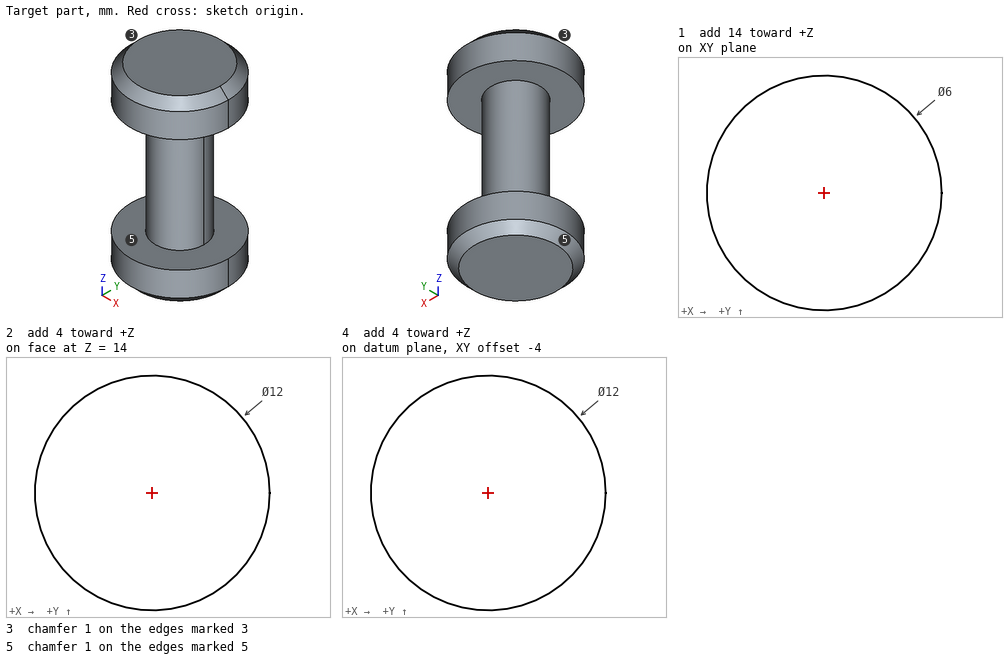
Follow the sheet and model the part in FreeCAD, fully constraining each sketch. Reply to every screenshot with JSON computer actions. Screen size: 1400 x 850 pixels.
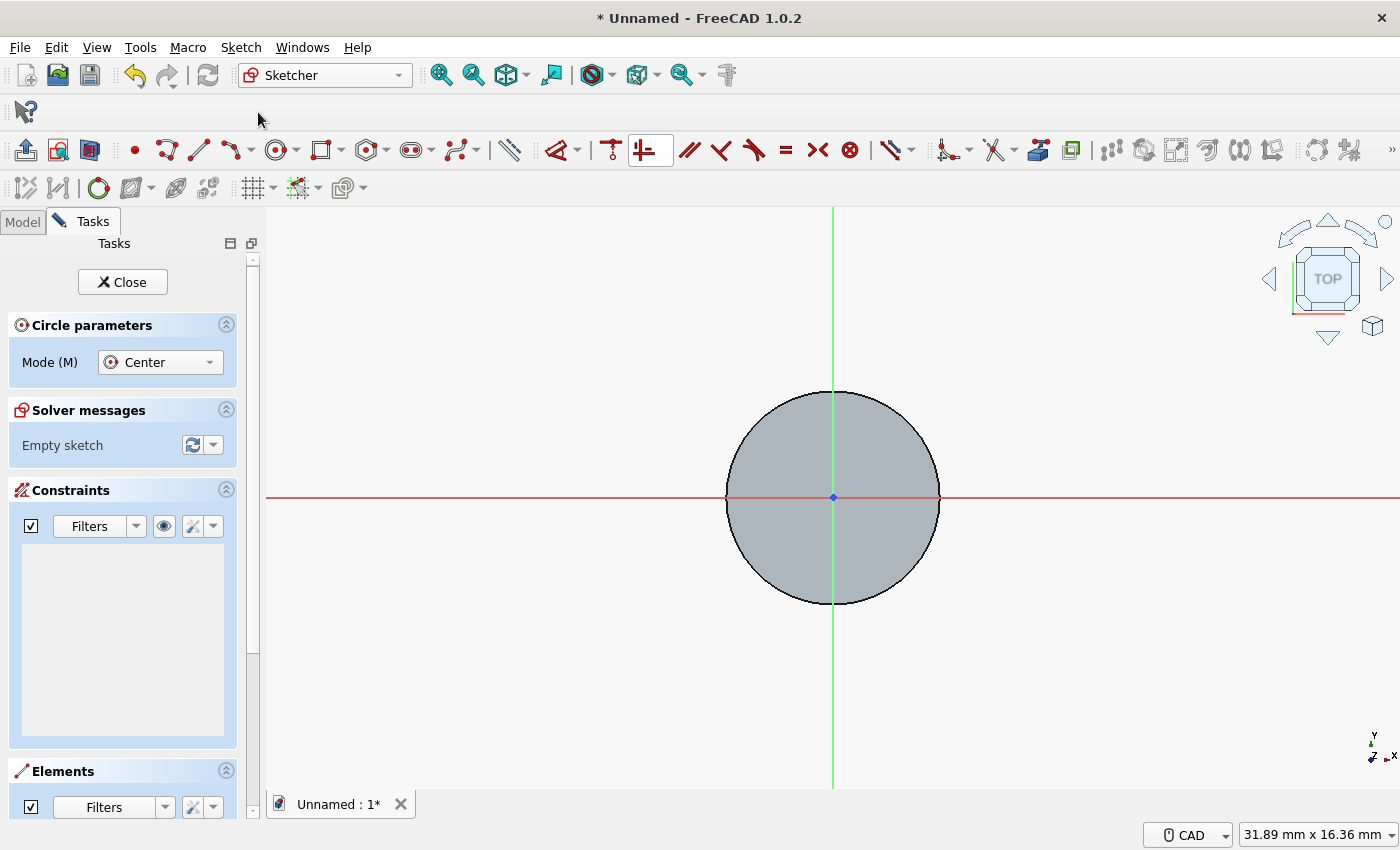
{"action": "left_click", "coordinate": [833, 498]}
{"action": "left_click", "coordinate": [984, 347]}
{"action": "key", "text": "Escape"}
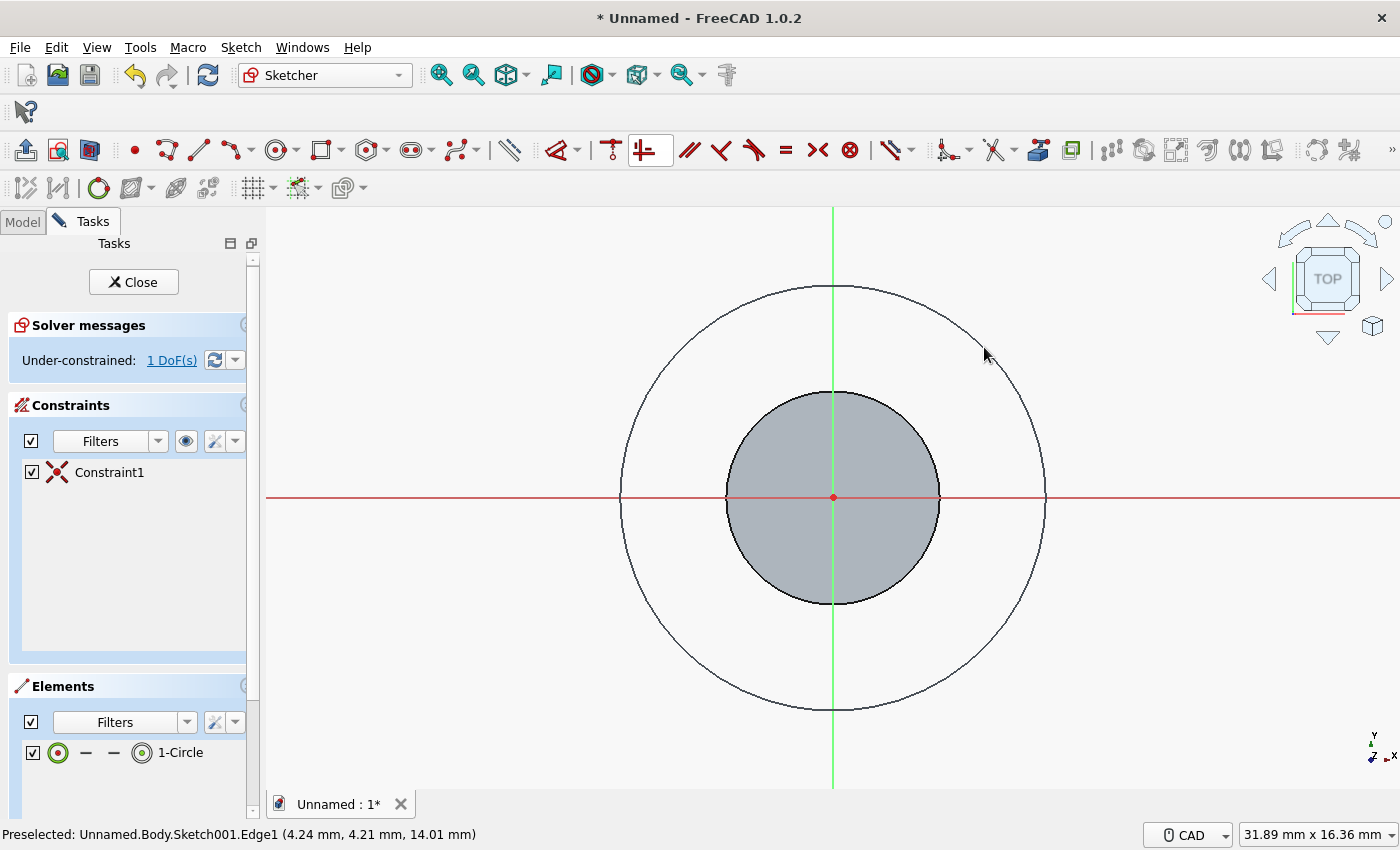
{"action": "left_click", "coordinate": [983, 347]}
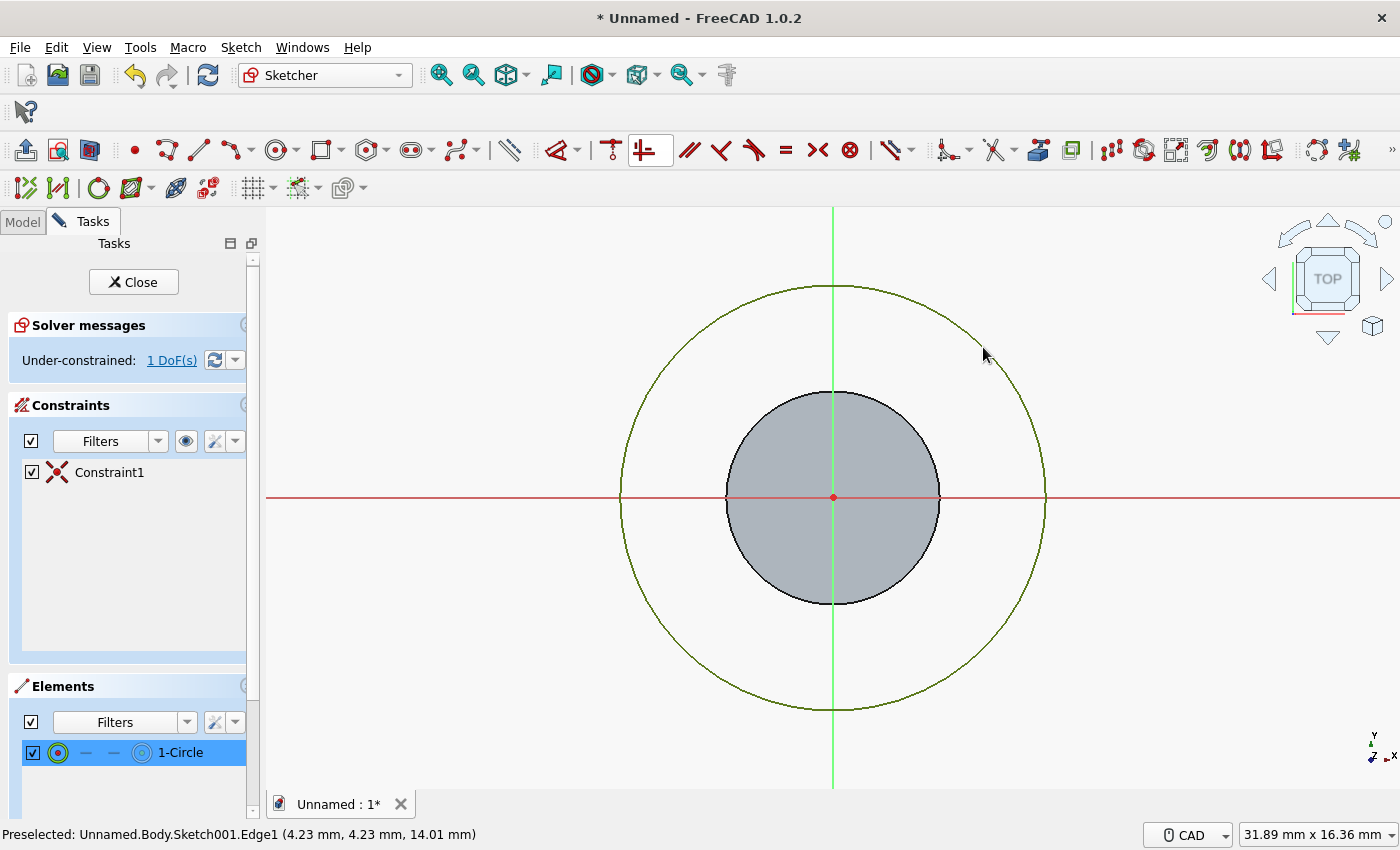
{"action": "key", "text": "k o"}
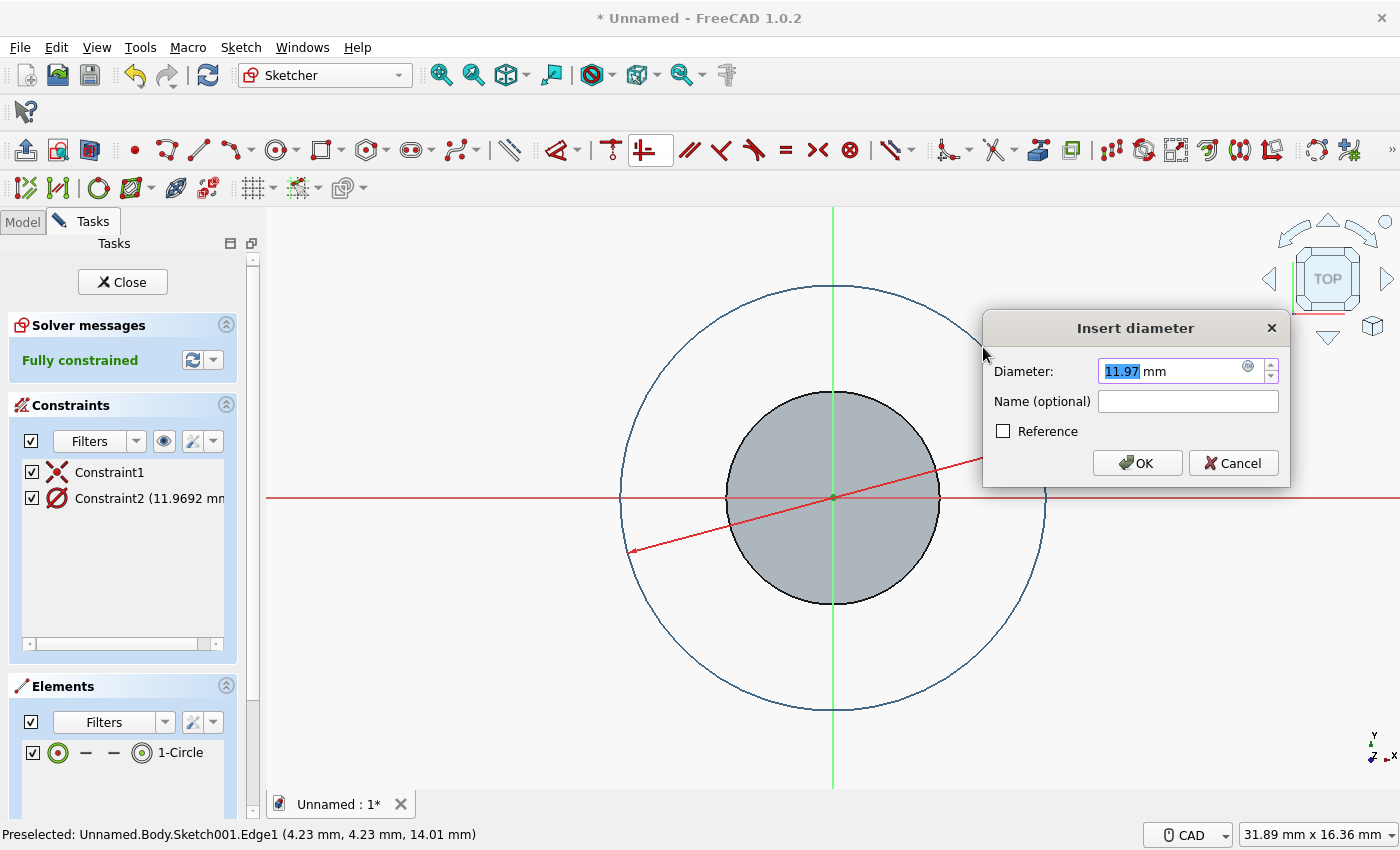
{"action": "type", "text": "12"}
{"action": "key", "text": "Return"}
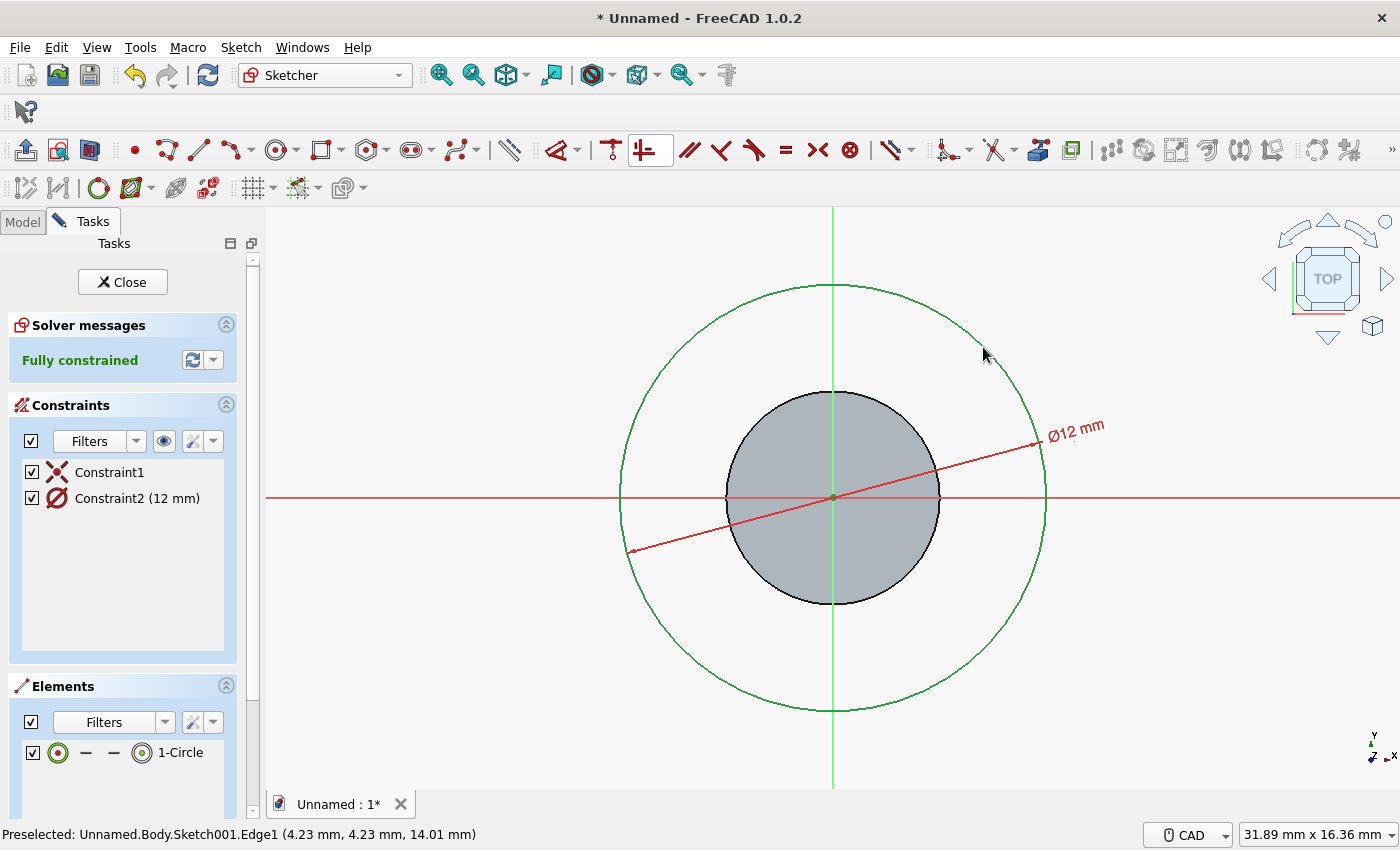
{"action": "left_click", "coordinate": [123, 282]}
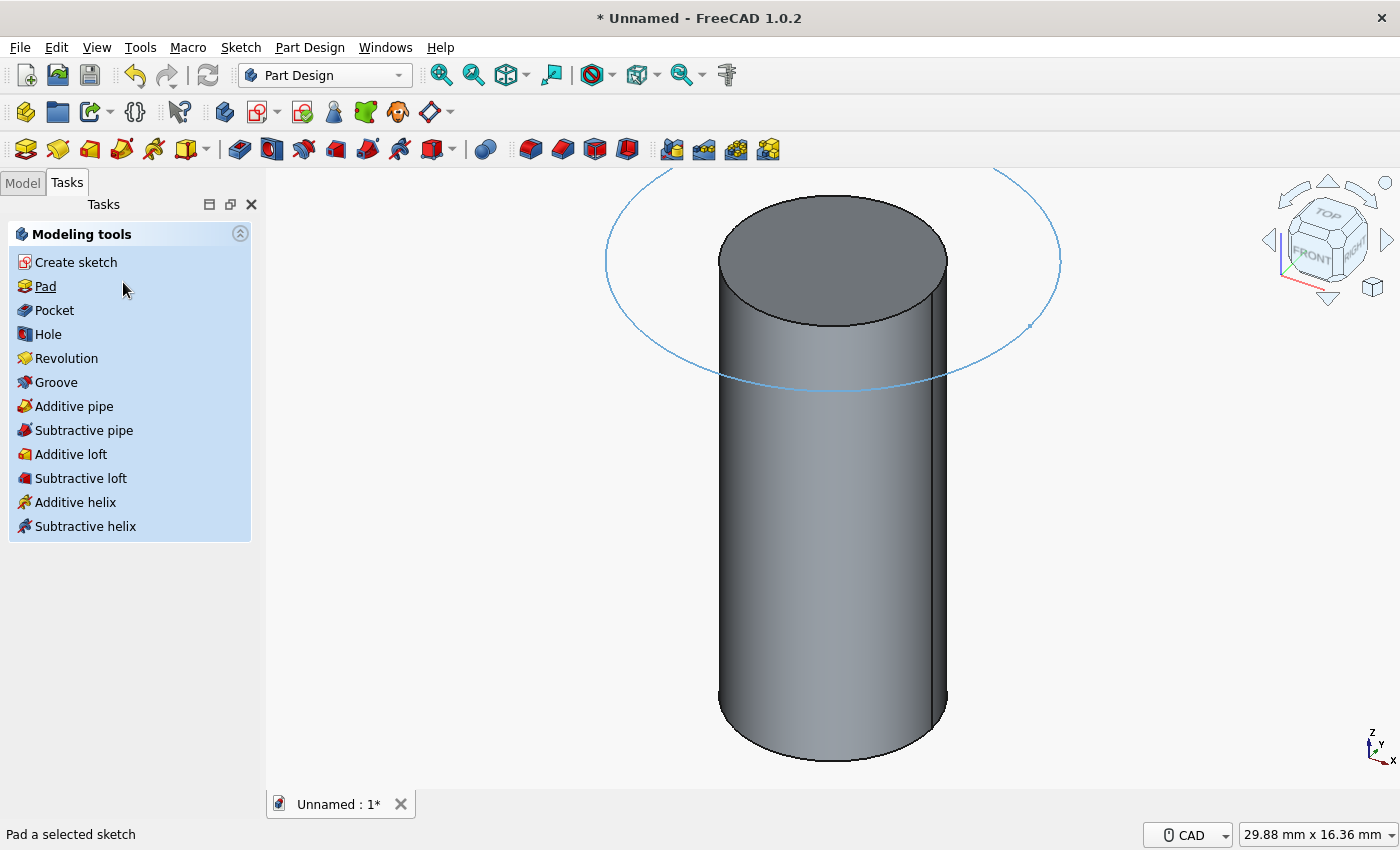
{"action": "left_click", "coordinate": [26, 150]}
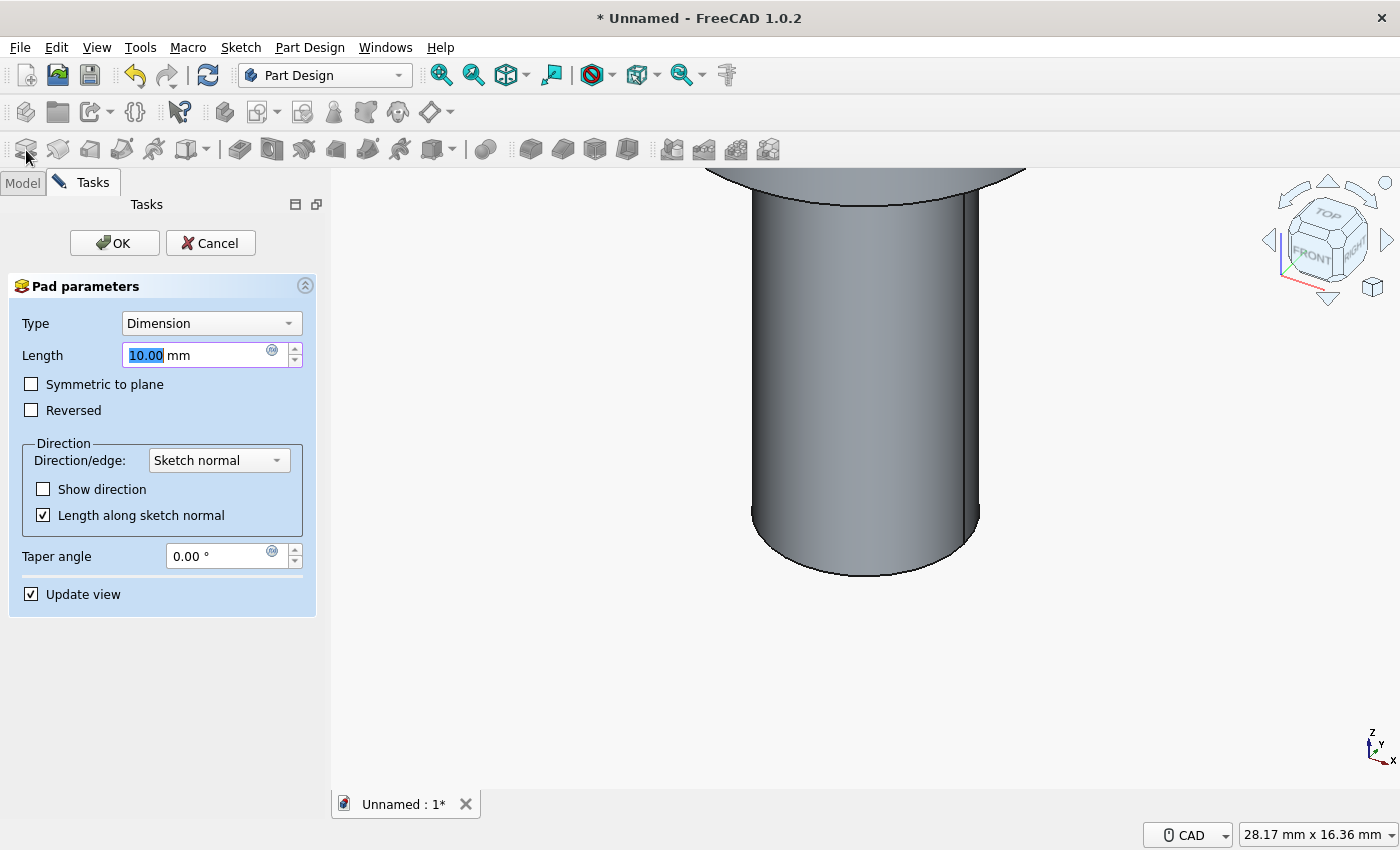
{"action": "type", "text": "4"}
{"action": "key", "text": "Tab"}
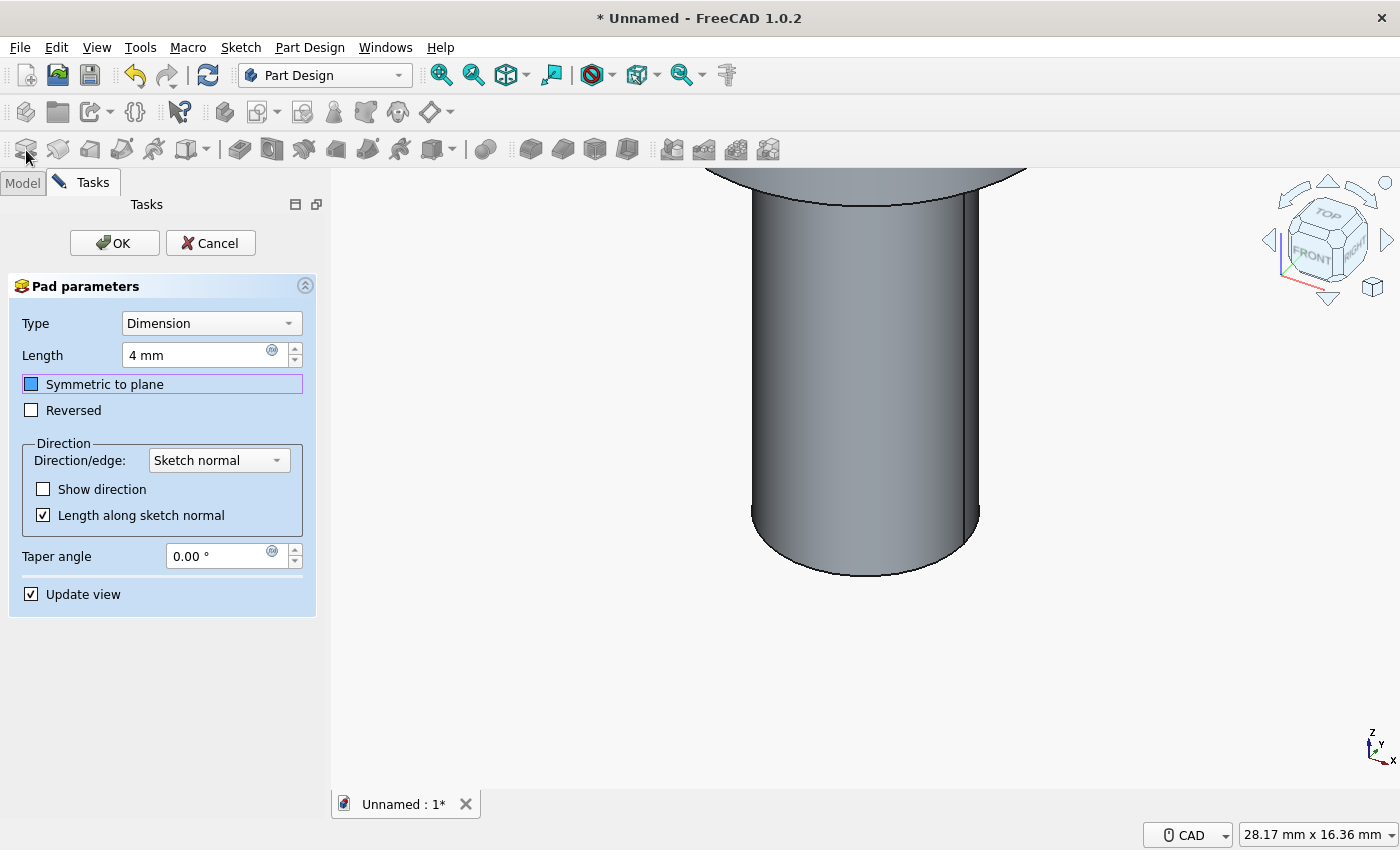
{"action": "left_click", "coordinate": [115, 243]}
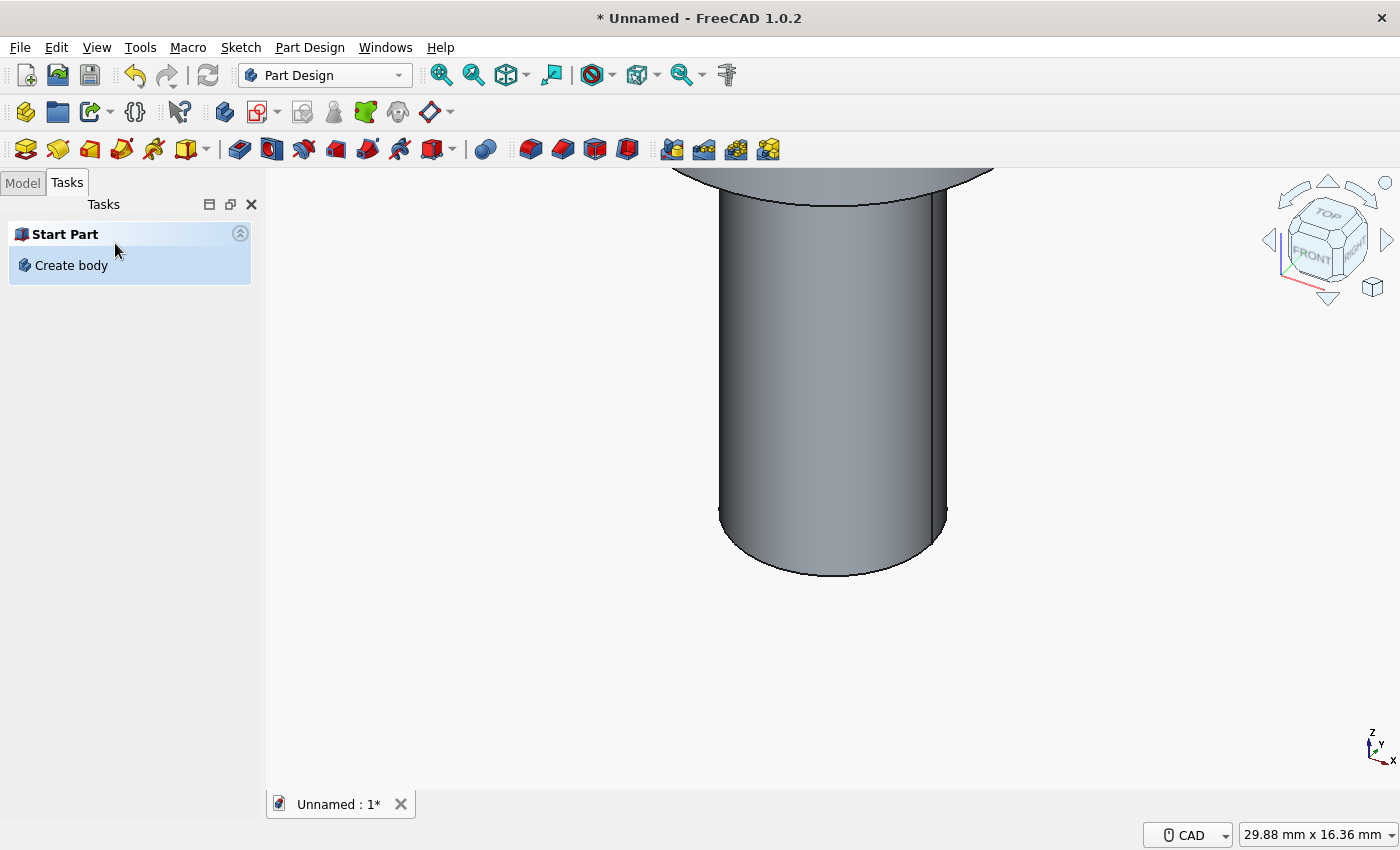
{"action": "key", "text": "v f"}